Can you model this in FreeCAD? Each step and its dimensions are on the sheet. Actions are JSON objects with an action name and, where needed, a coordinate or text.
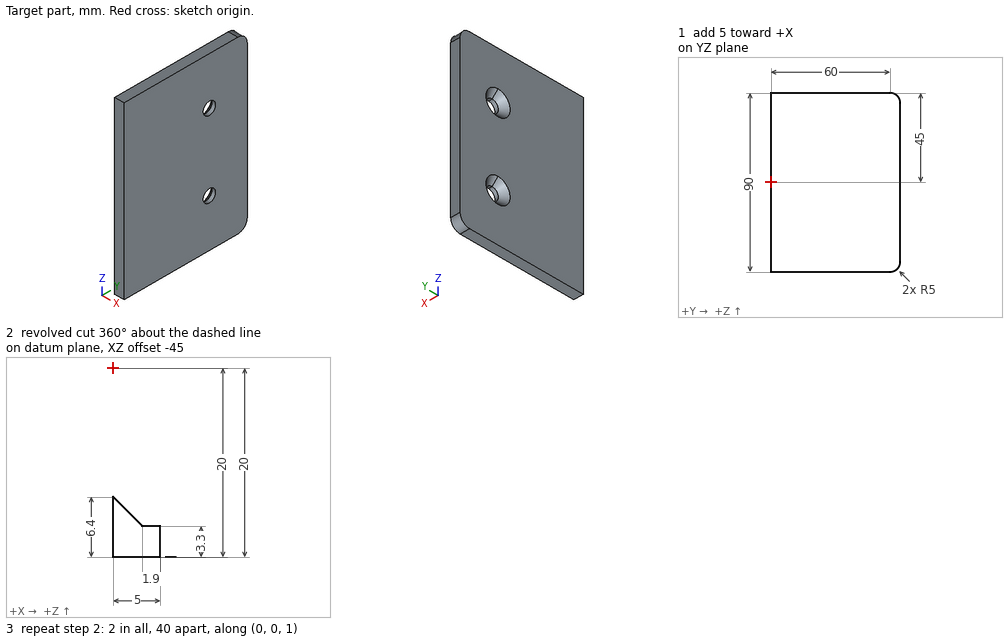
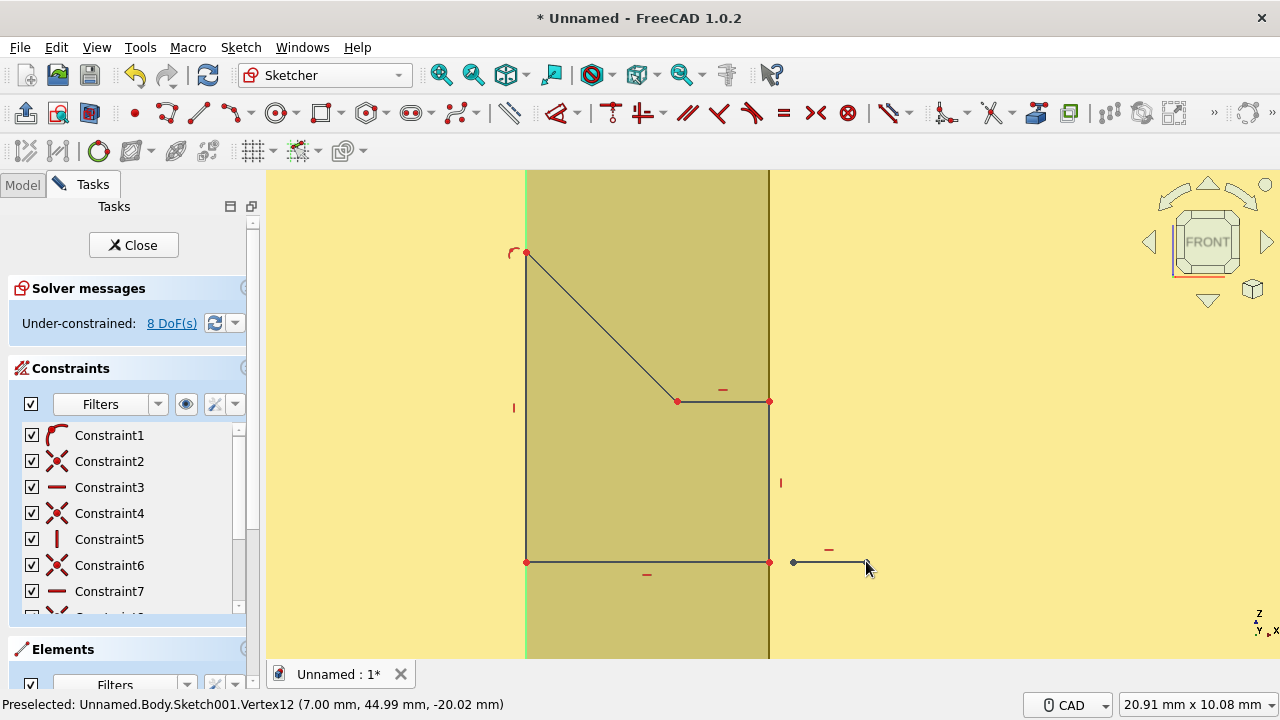
{"action": "left_click", "coordinate": [815, 562]}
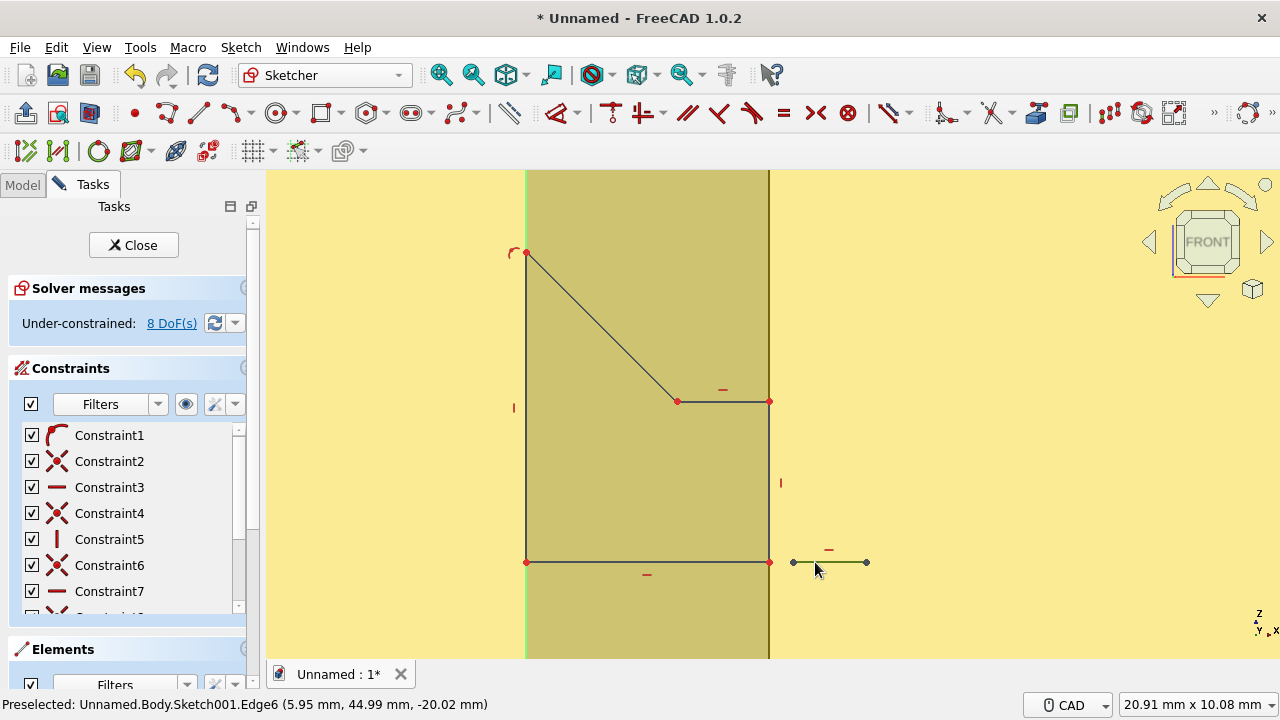
{"action": "left_click", "coordinate": [510, 114]}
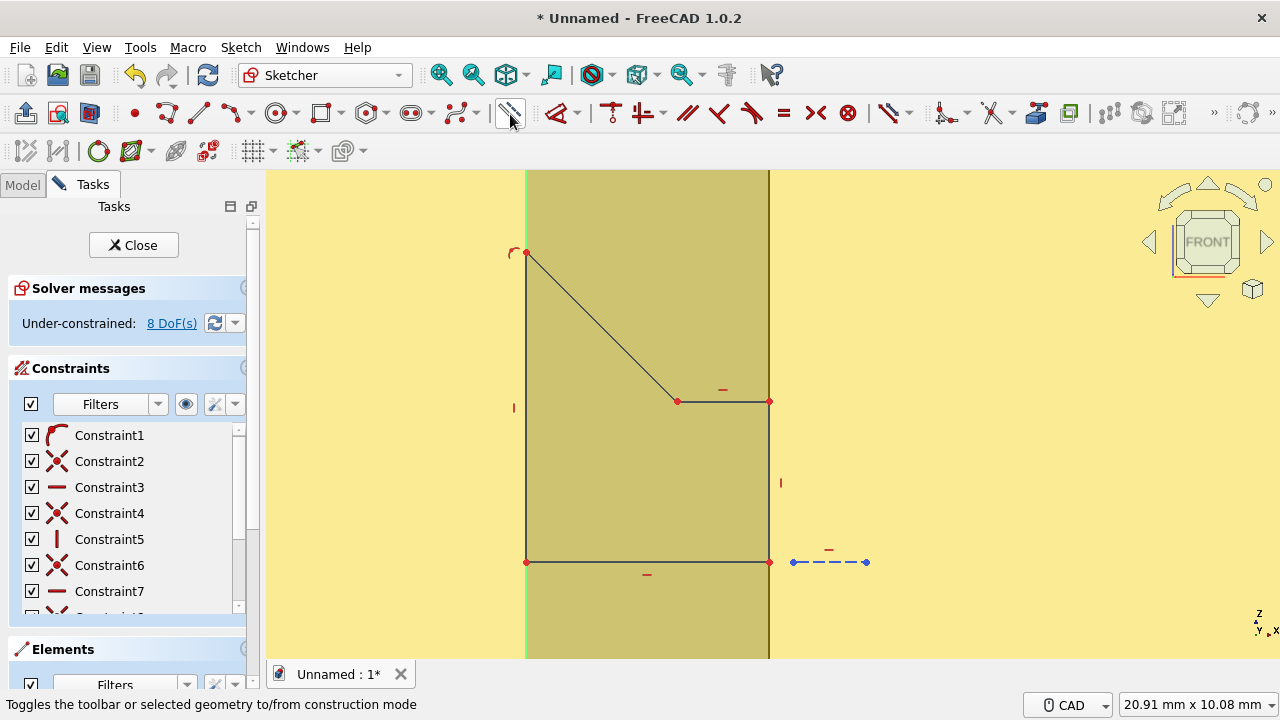
{"action": "left_click", "coordinate": [556, 114]}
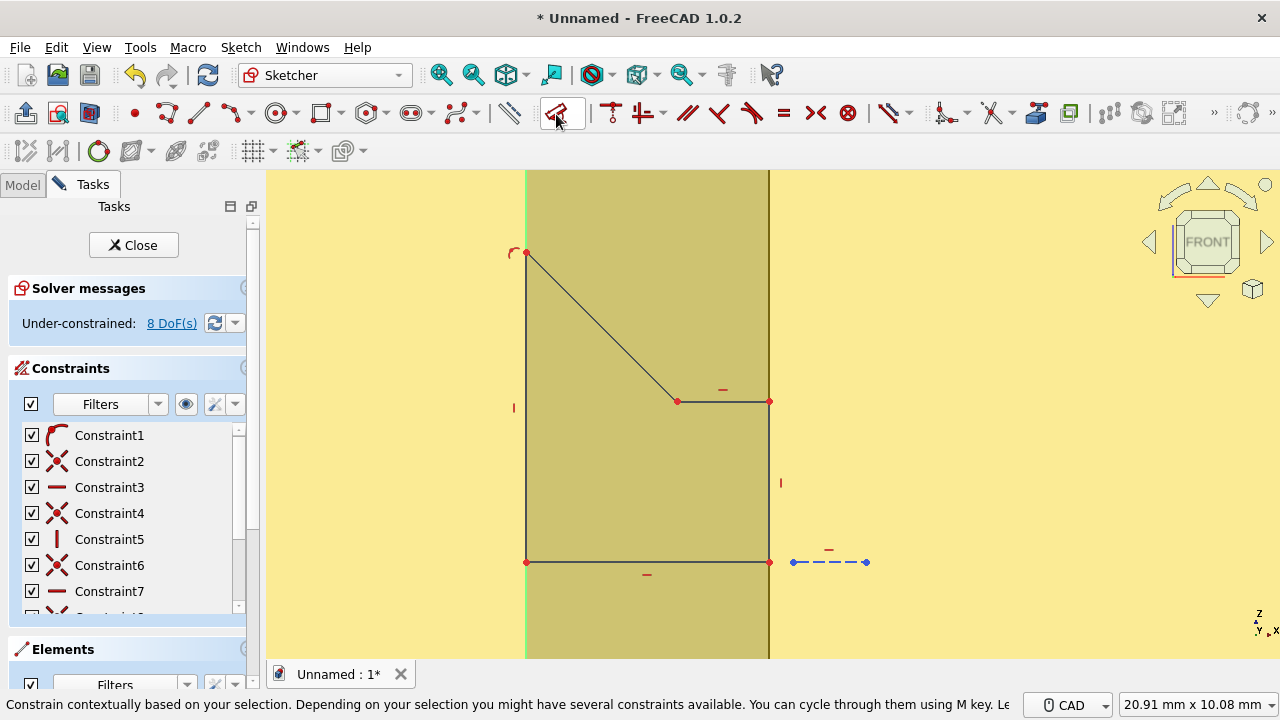
{"action": "left_click", "coordinate": [696, 562]}
{"action": "left_click", "coordinate": [648, 596]}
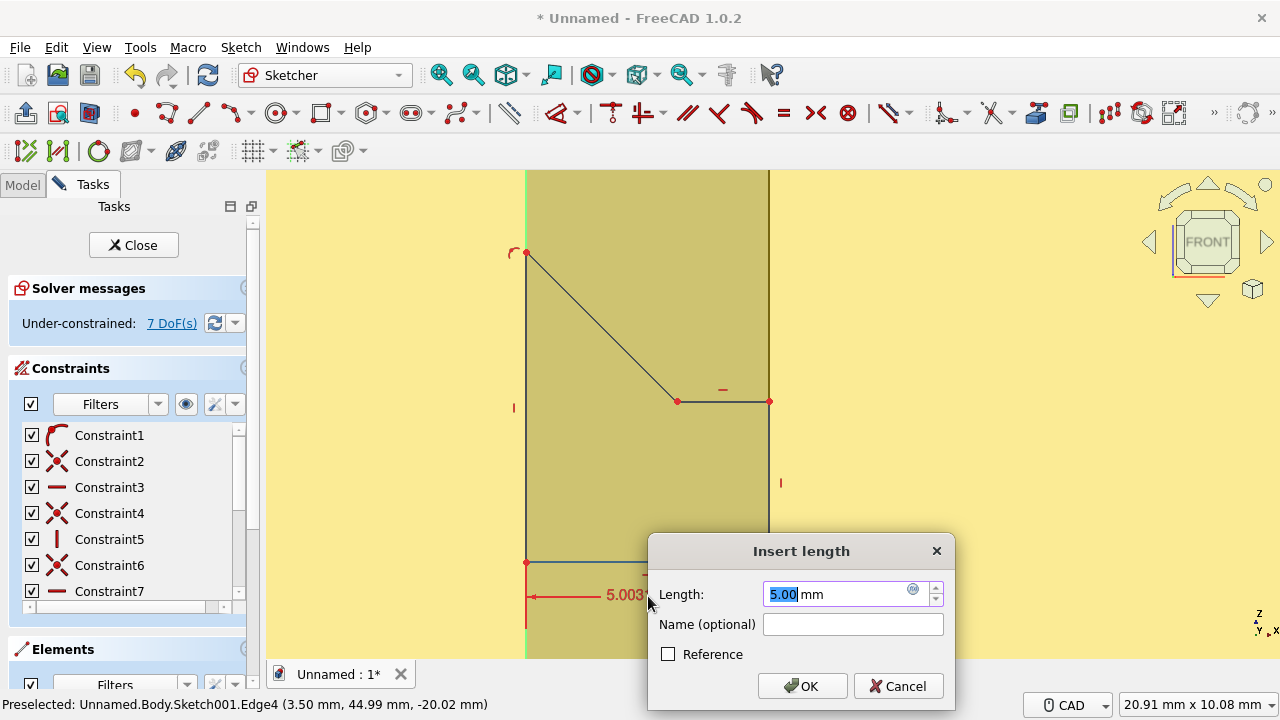
{"action": "type", "text": "5"}
{"action": "key", "text": "Return"}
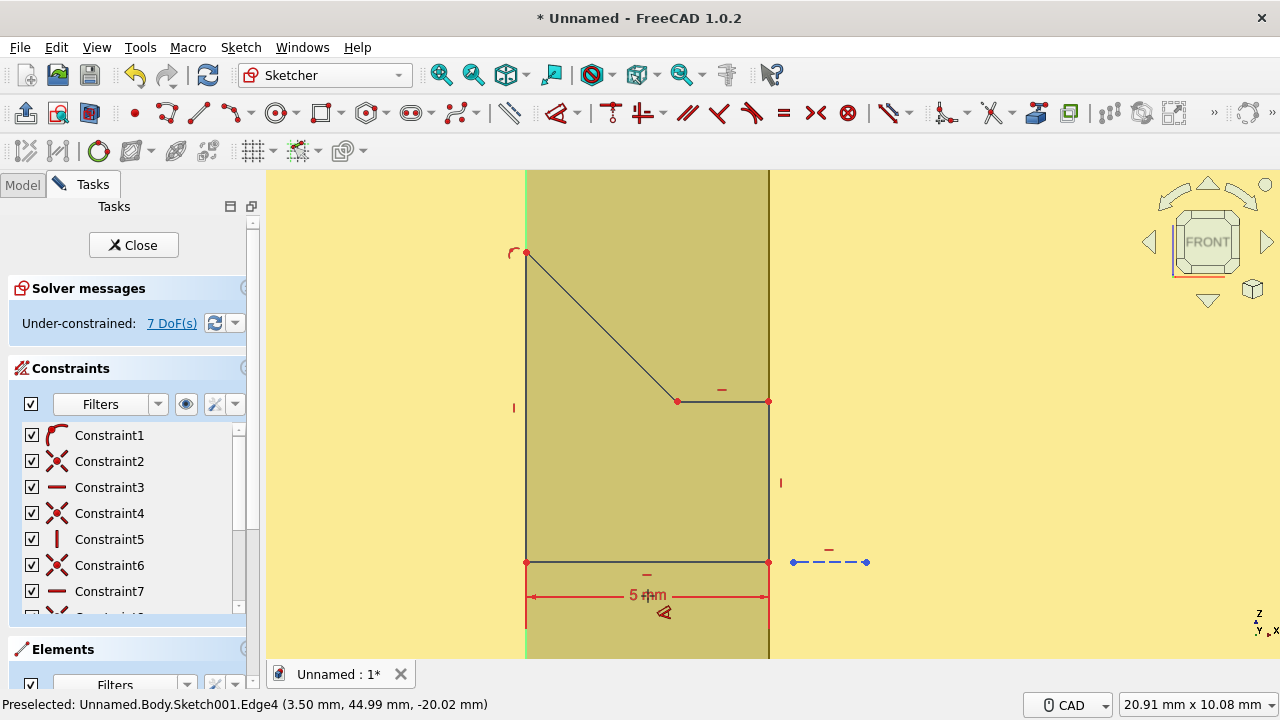
{"action": "left_click", "coordinate": [705, 402]}
{"action": "left_click", "coordinate": [723, 368]}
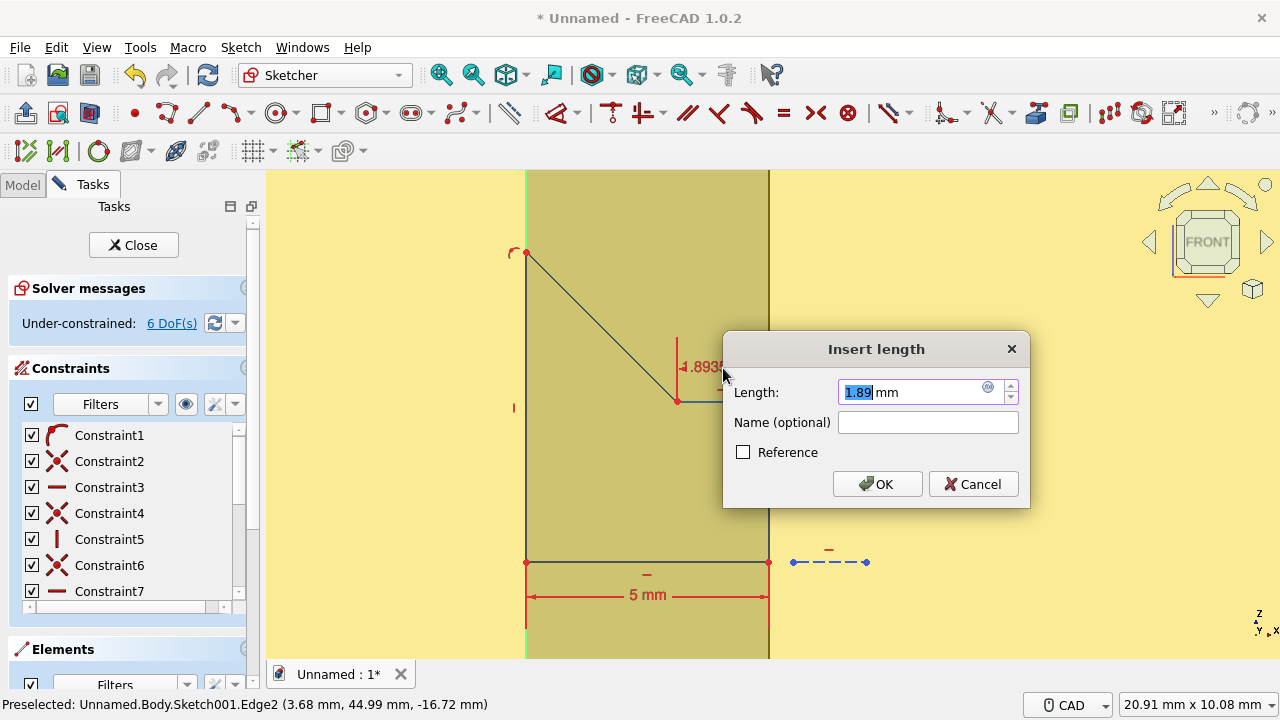
{"action": "type", "text": "1.9"}
{"action": "key", "text": "Return"}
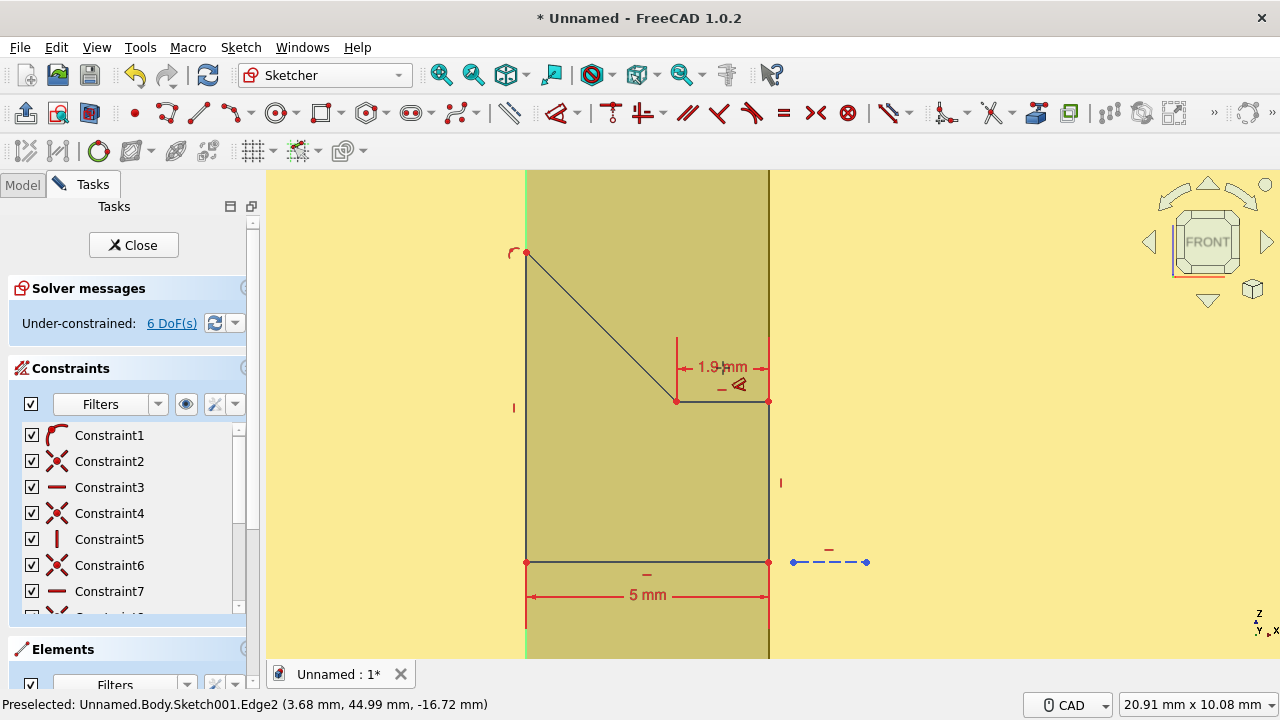
{"action": "left_click", "coordinate": [769, 450]}
{"action": "left_click", "coordinate": [803, 482]}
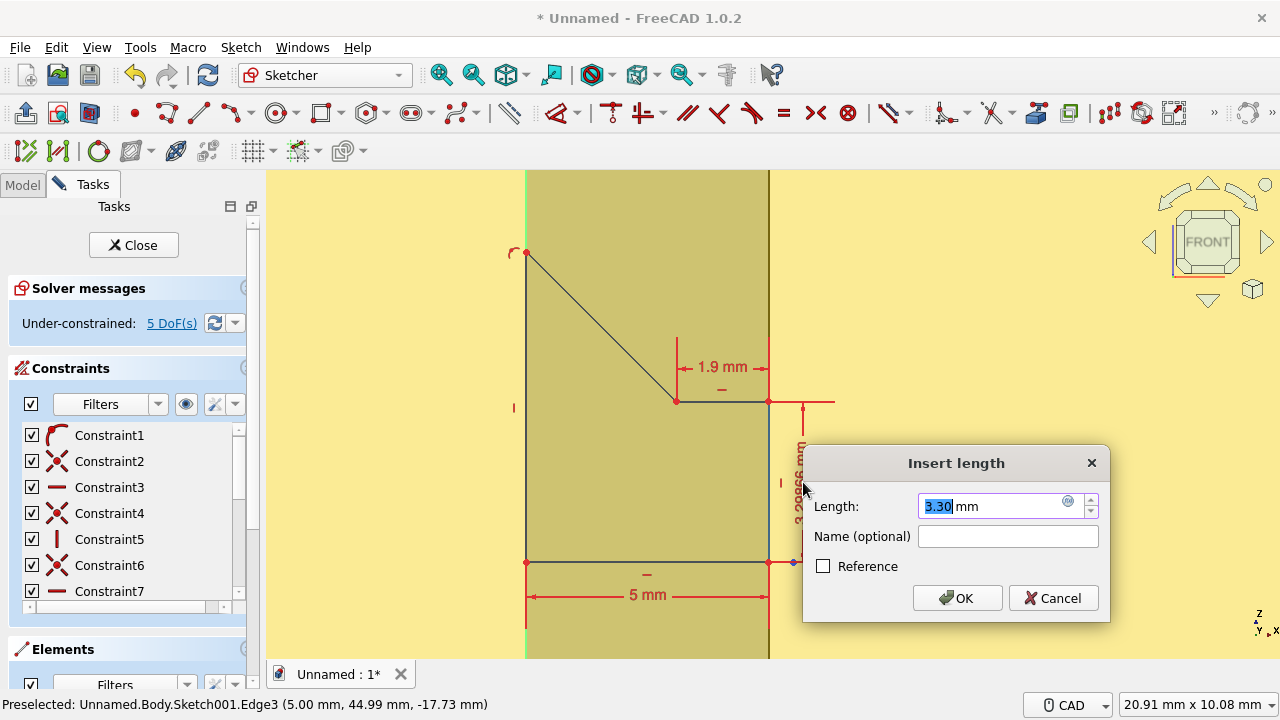
{"action": "type", "text": "3.3"}
{"action": "key", "text": "Return"}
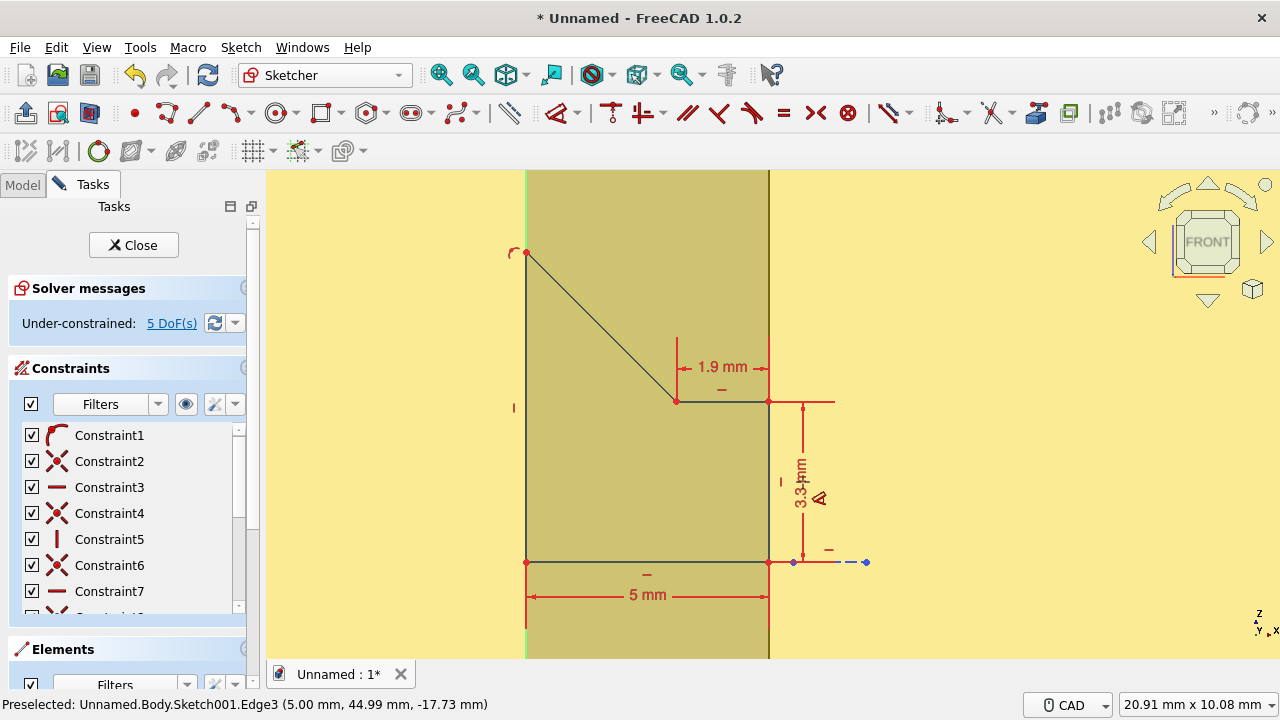
{"action": "left_click", "coordinate": [526, 469]}
{"action": "left_click", "coordinate": [492, 407]}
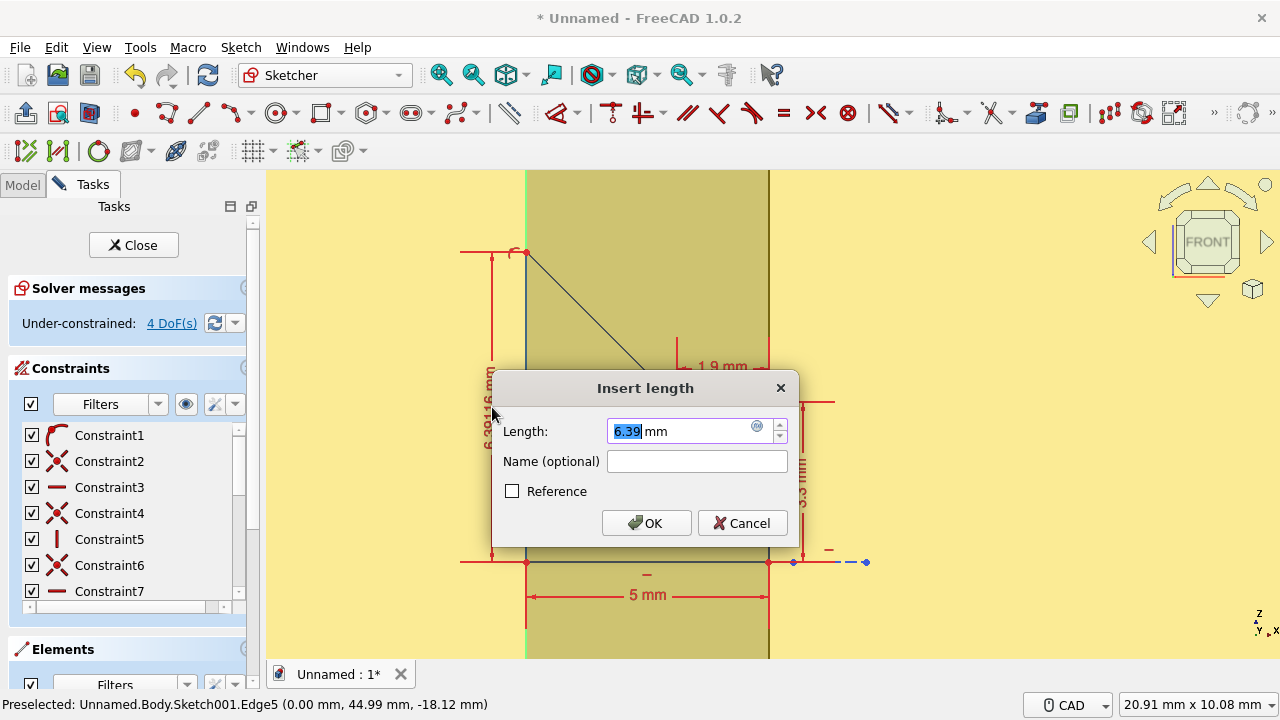
{"action": "type", "text": "6.4"}
{"action": "key", "text": "Return"}